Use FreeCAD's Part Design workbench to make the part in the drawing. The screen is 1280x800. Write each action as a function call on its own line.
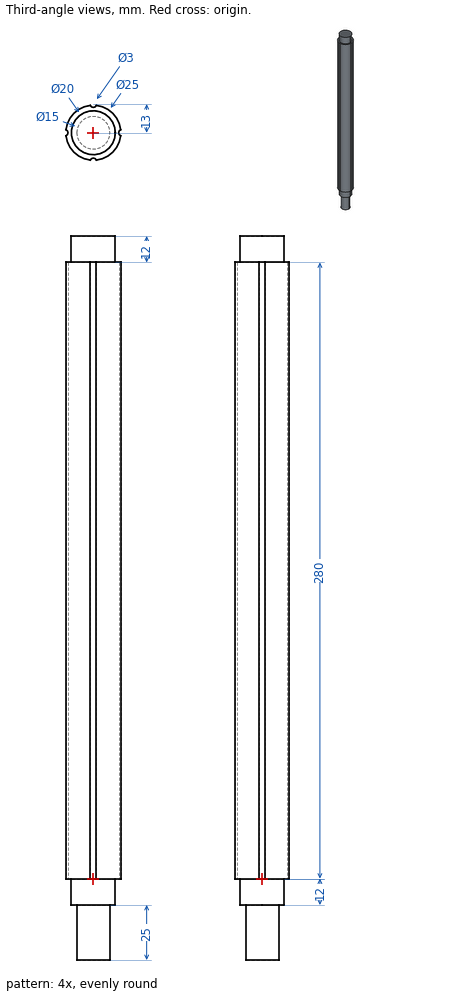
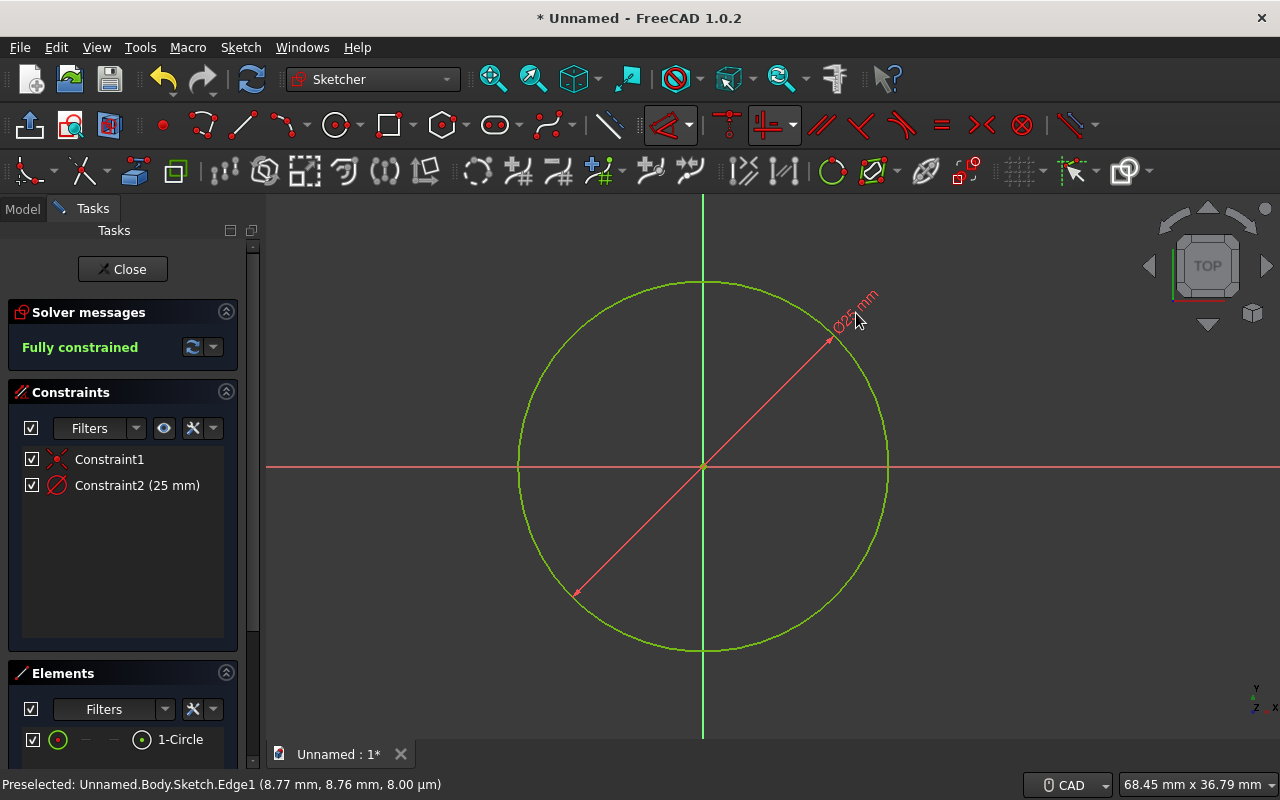
click(123, 269)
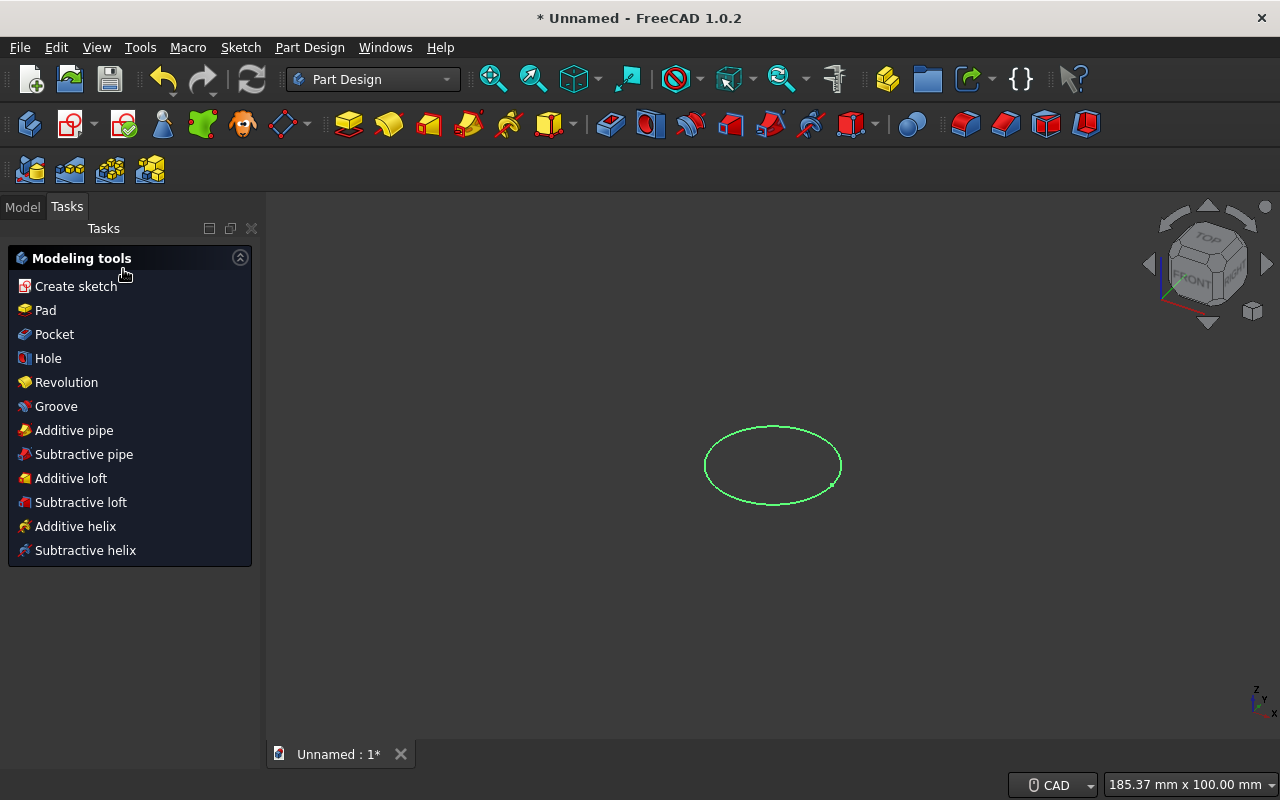
click(350, 124)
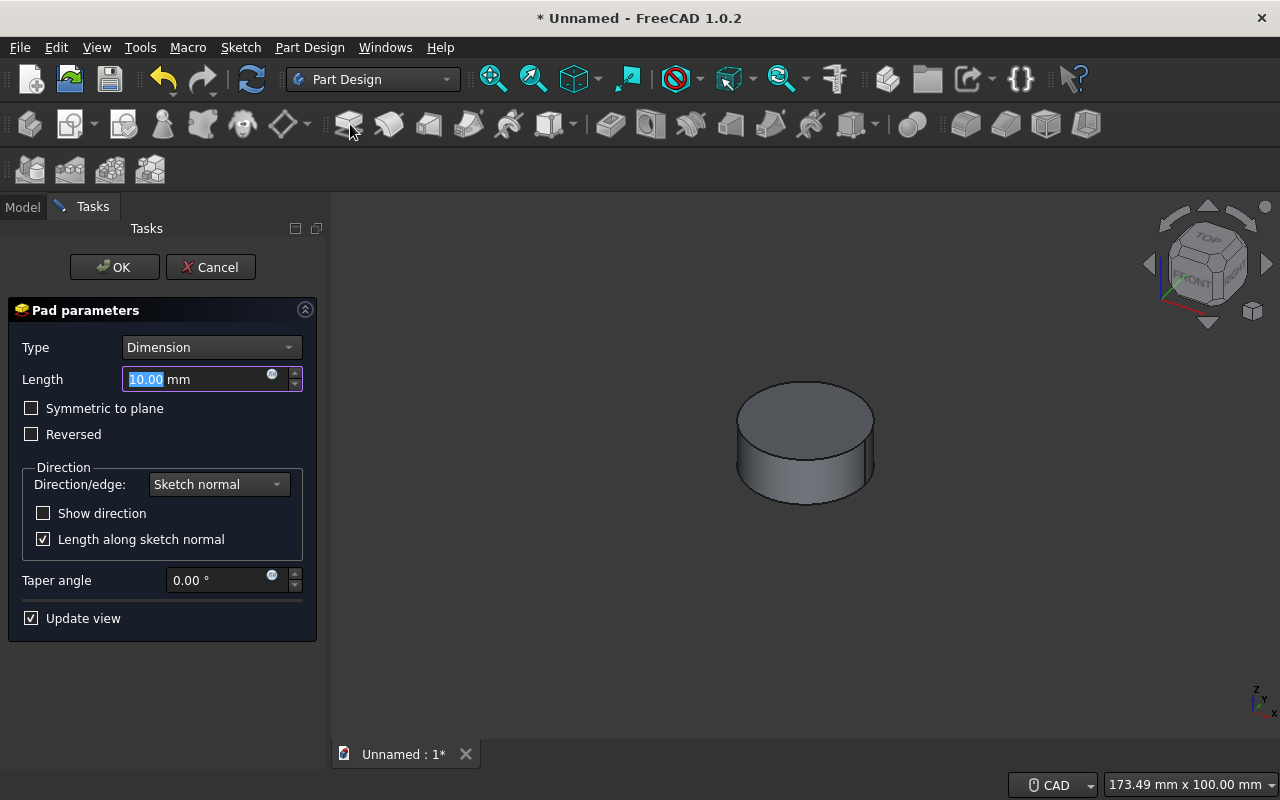
text(280)
key(Tab)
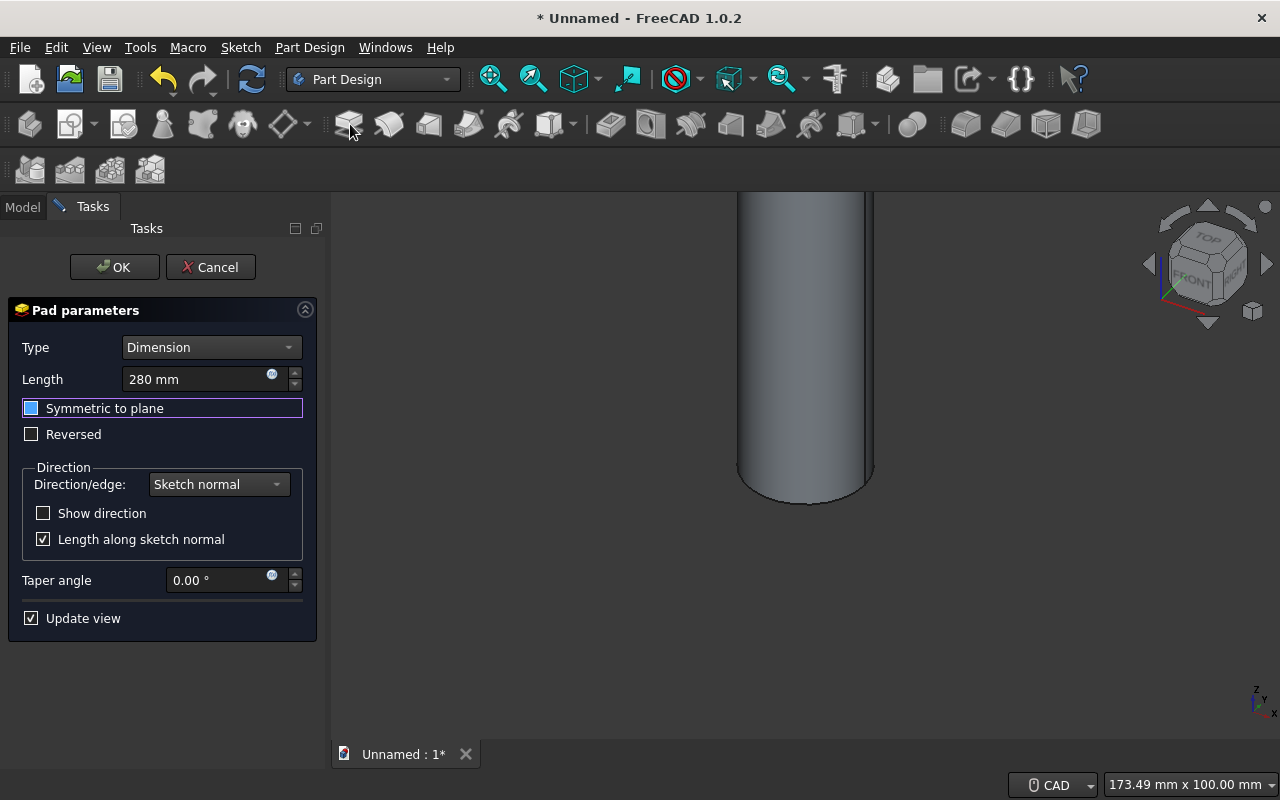
click(115, 267)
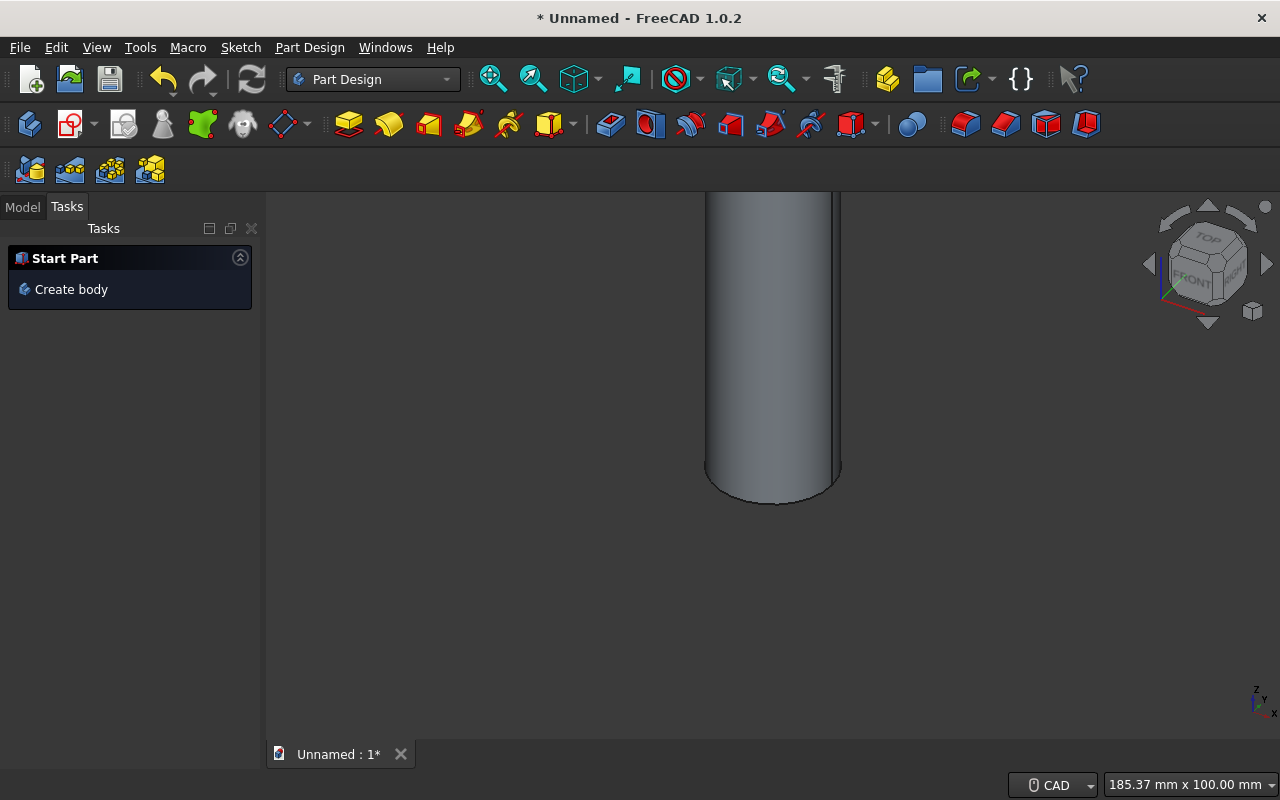
click(494, 80)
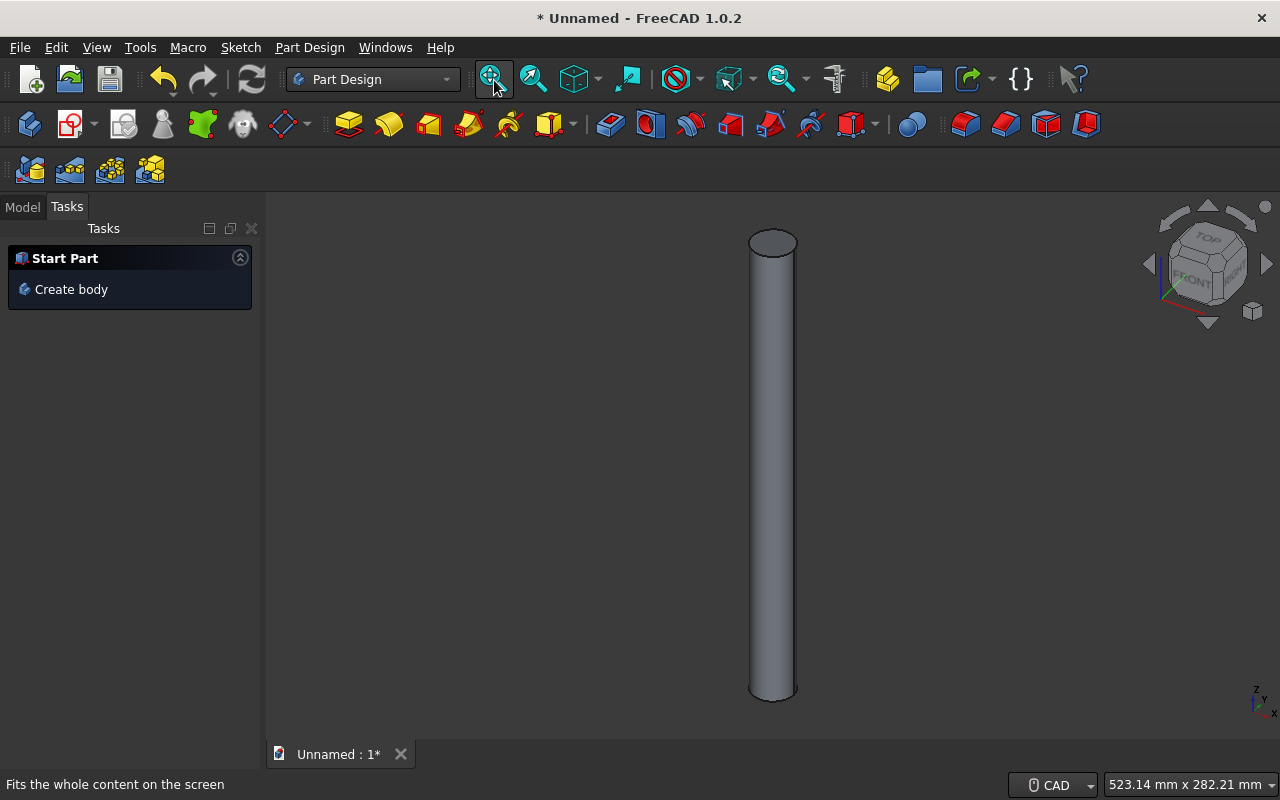
click(773, 242)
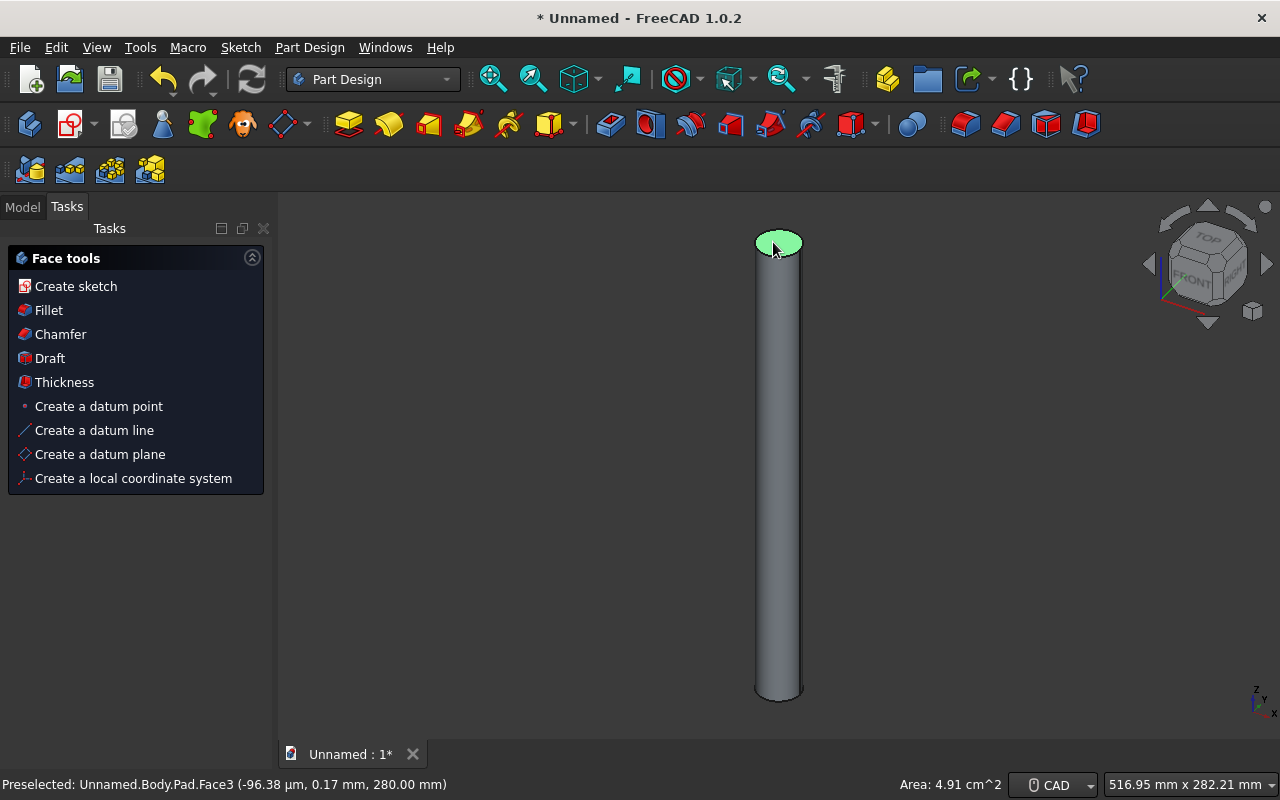
click(70, 124)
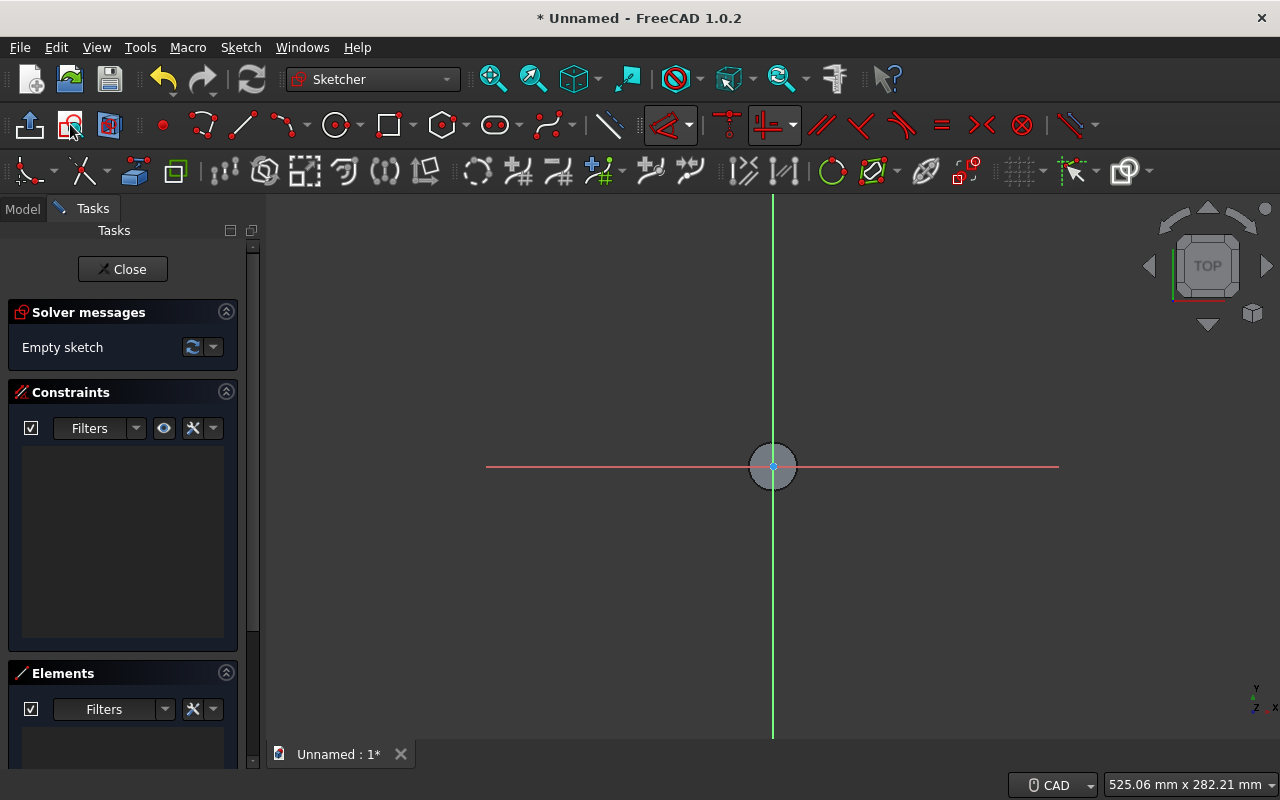
scroll(782, 466, up, 11)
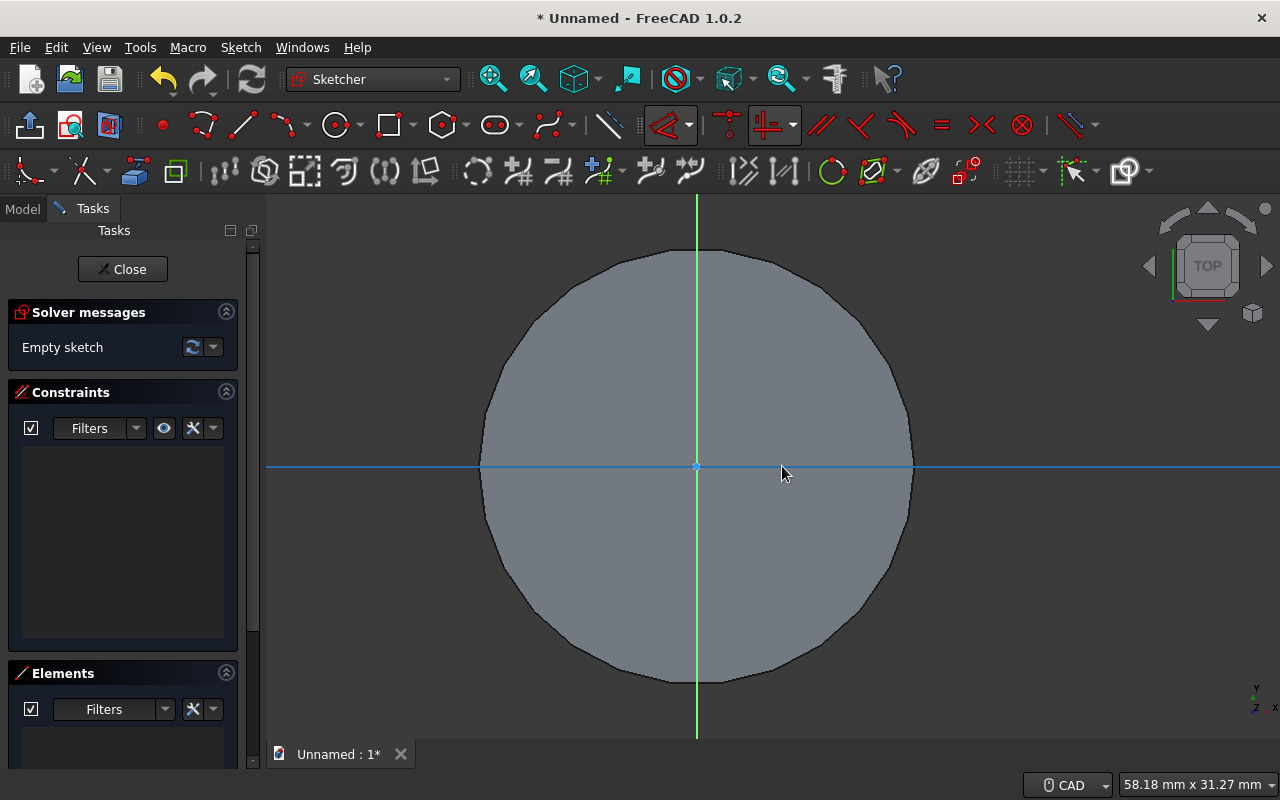
click(336, 126)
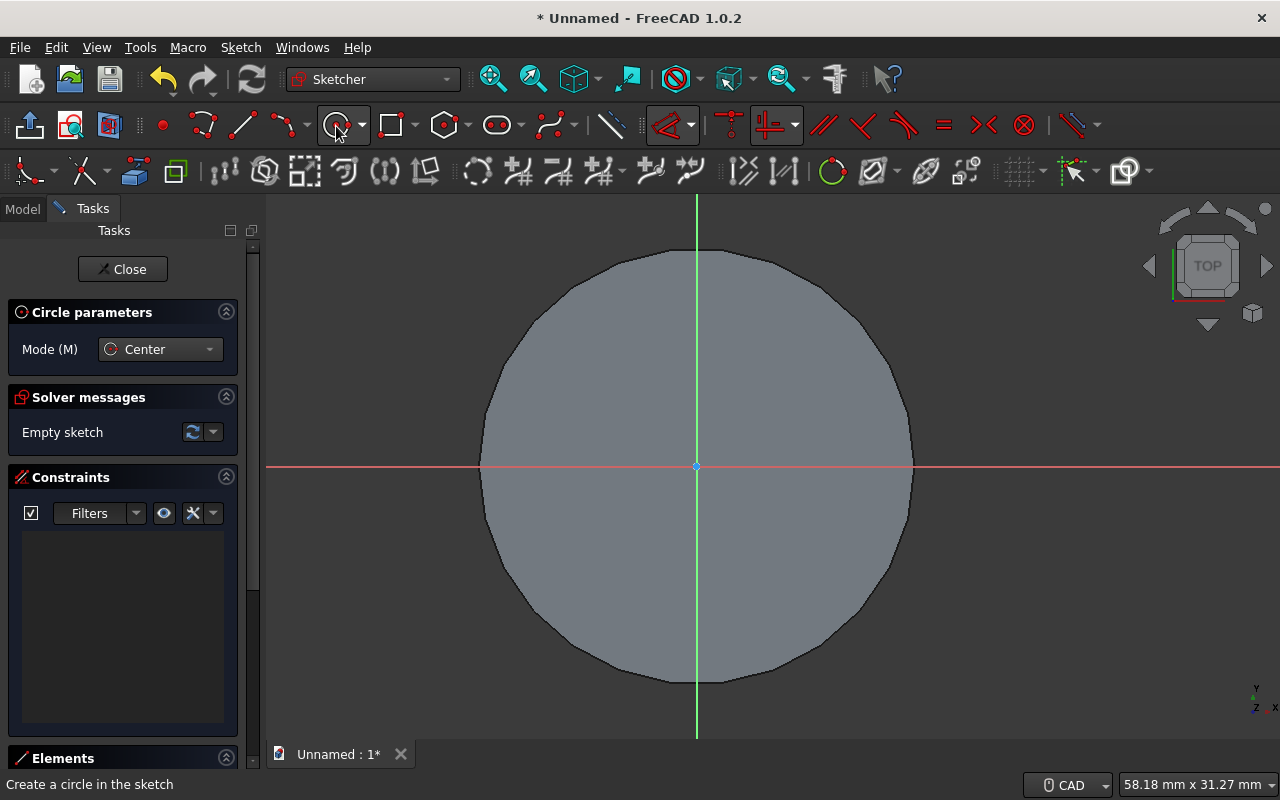
click(697, 466)
click(820, 343)
key(Escape)